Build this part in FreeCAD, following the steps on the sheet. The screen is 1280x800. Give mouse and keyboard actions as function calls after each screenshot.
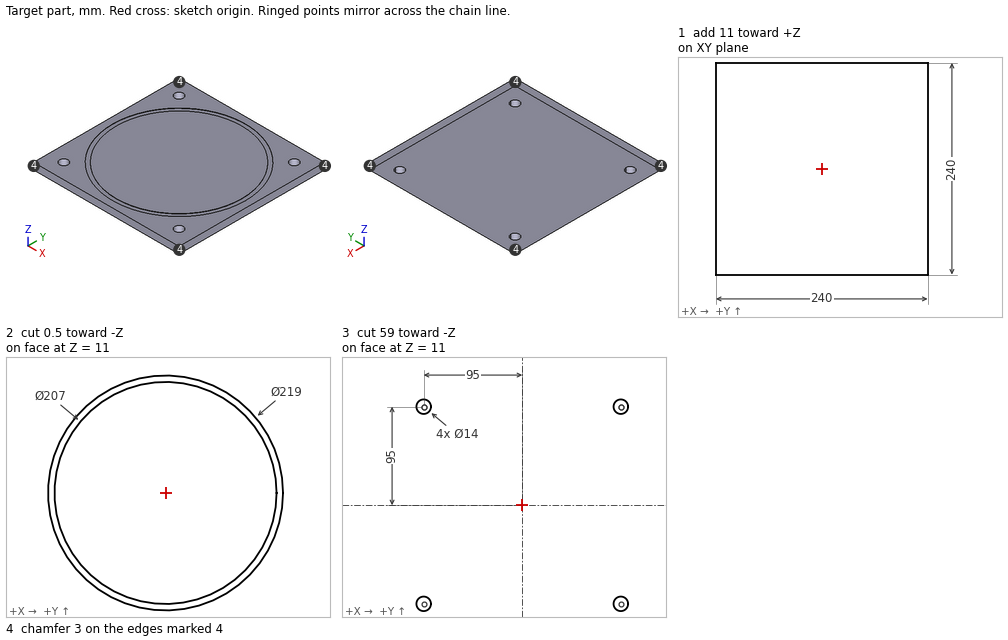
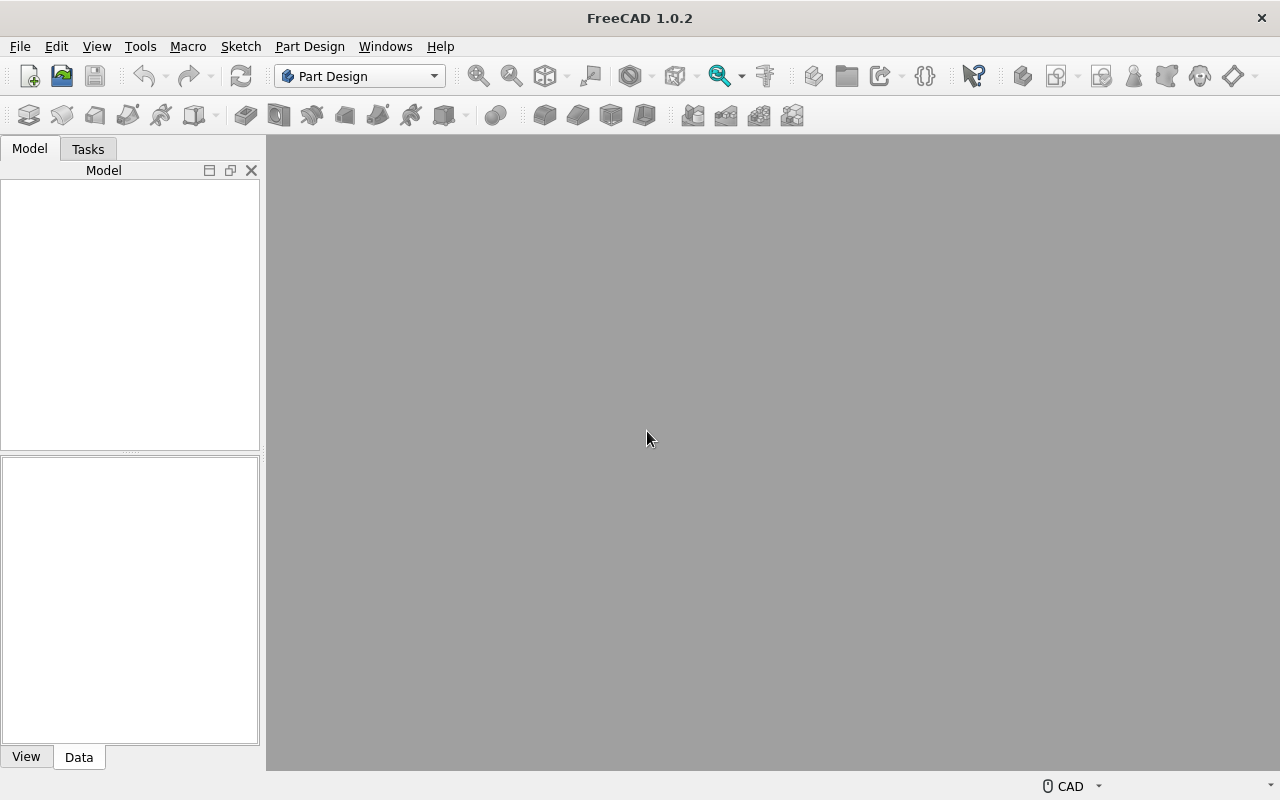
click(29, 76)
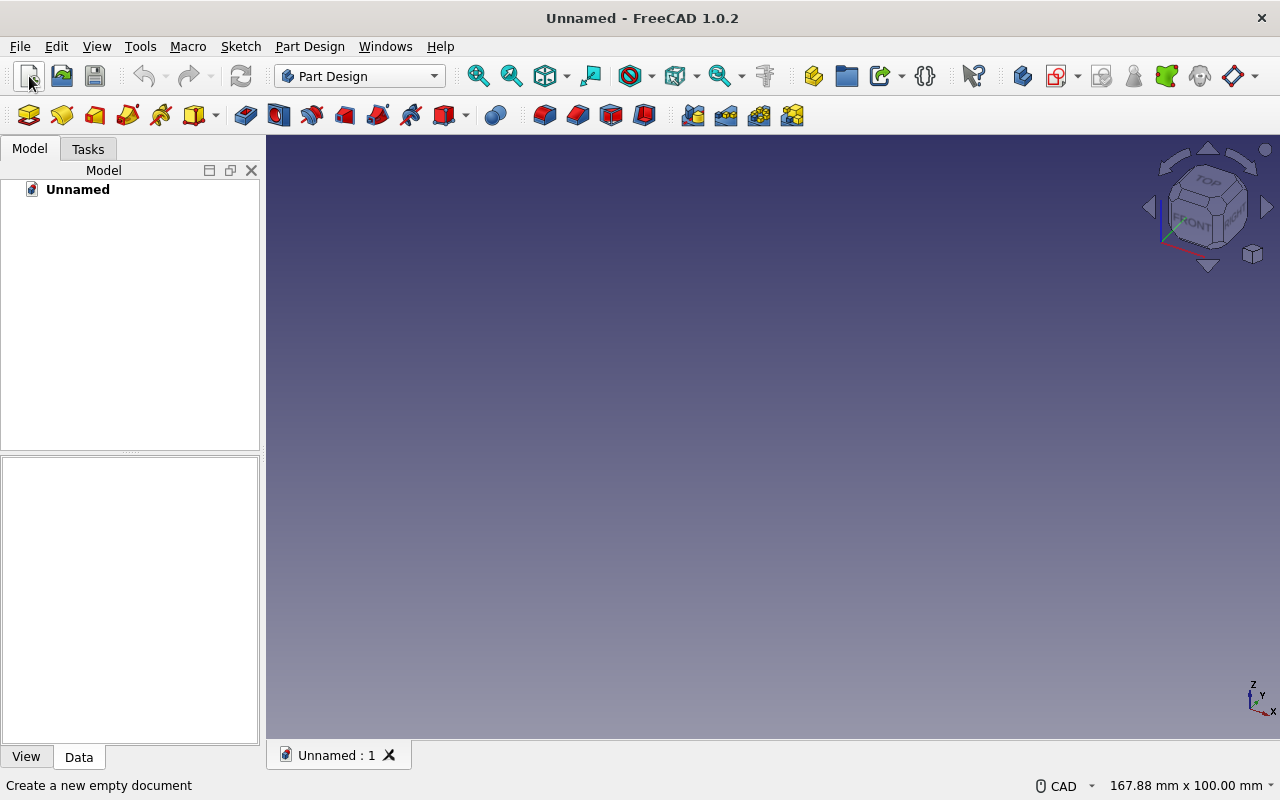
click(1056, 76)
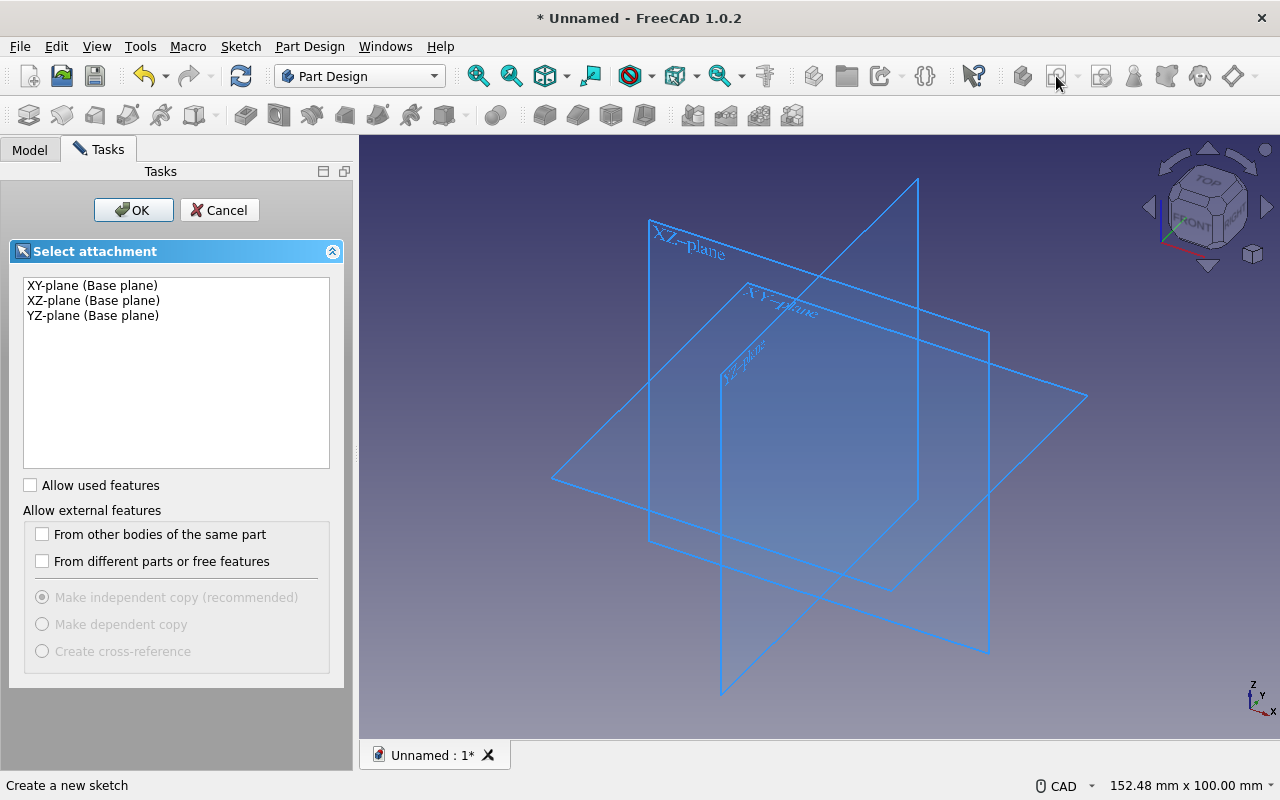
click(84, 286)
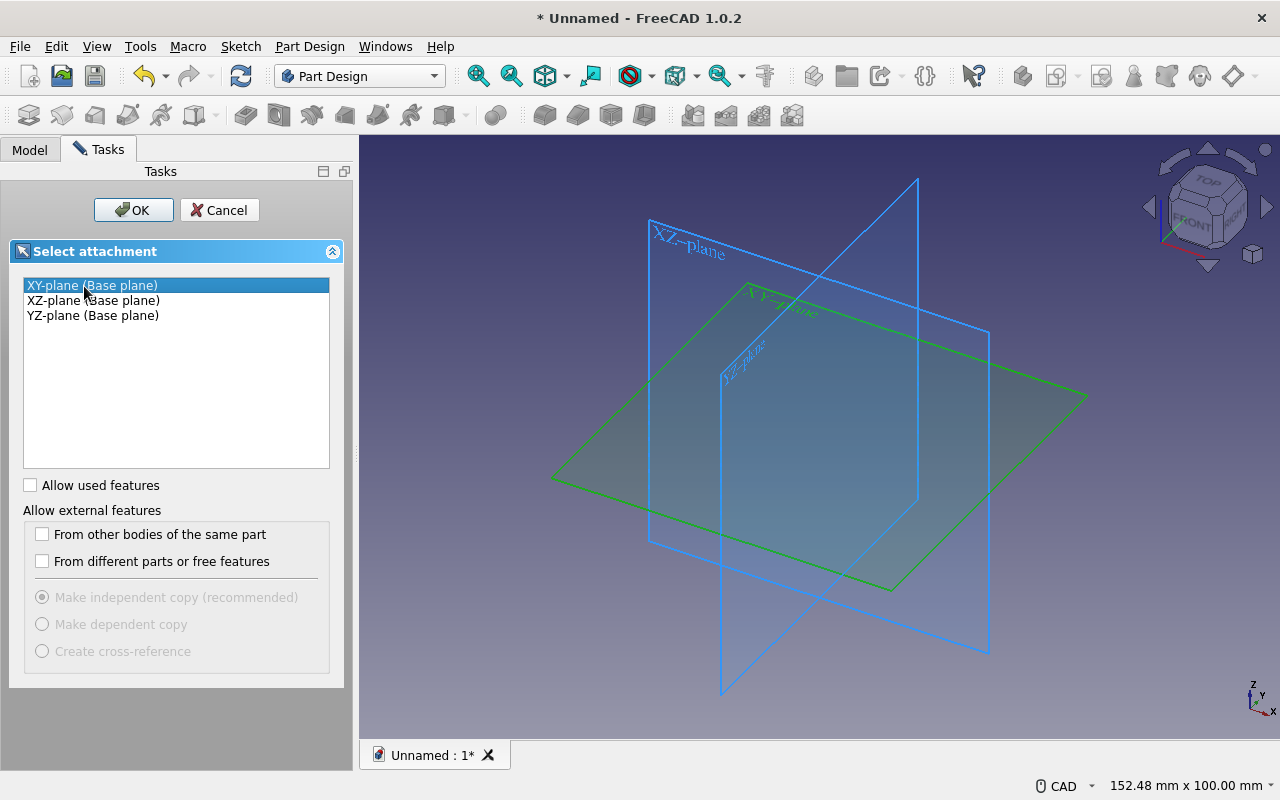
click(134, 210)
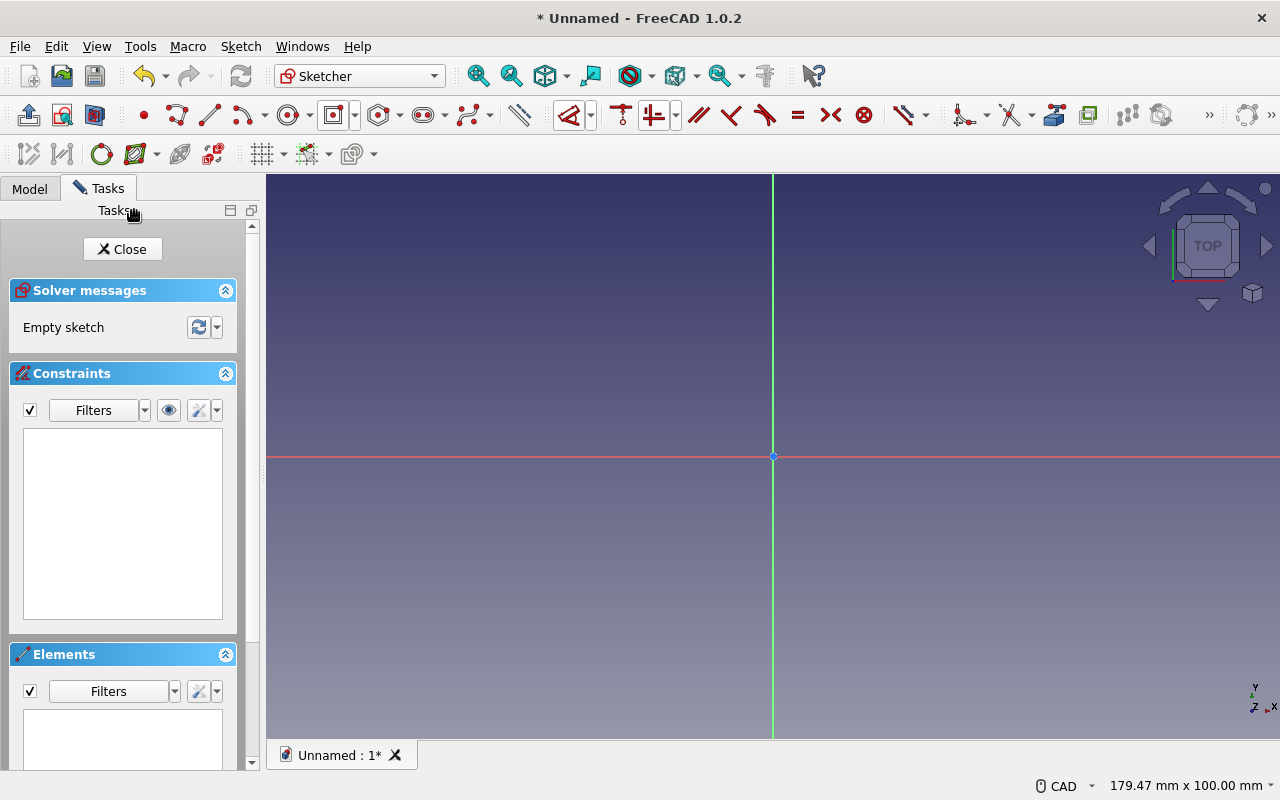
scroll(682, 456, down, 7)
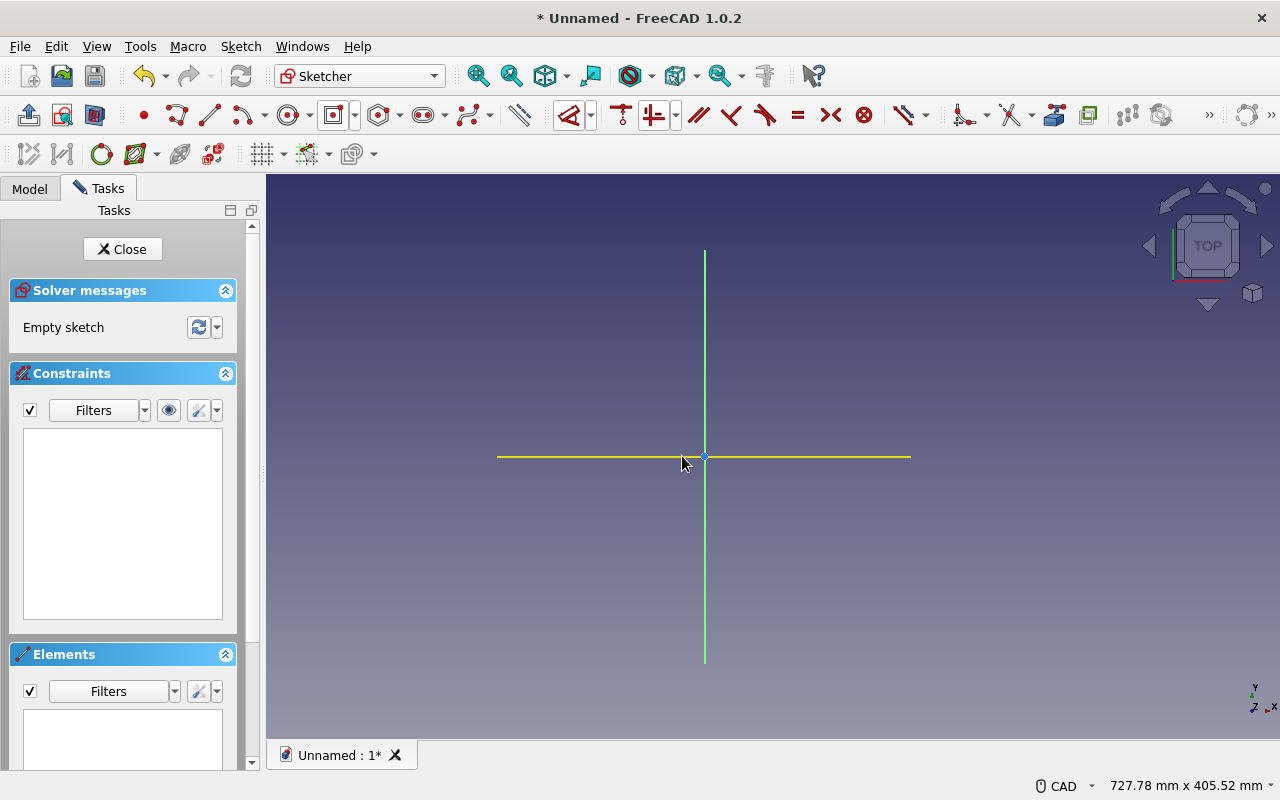
click(332, 116)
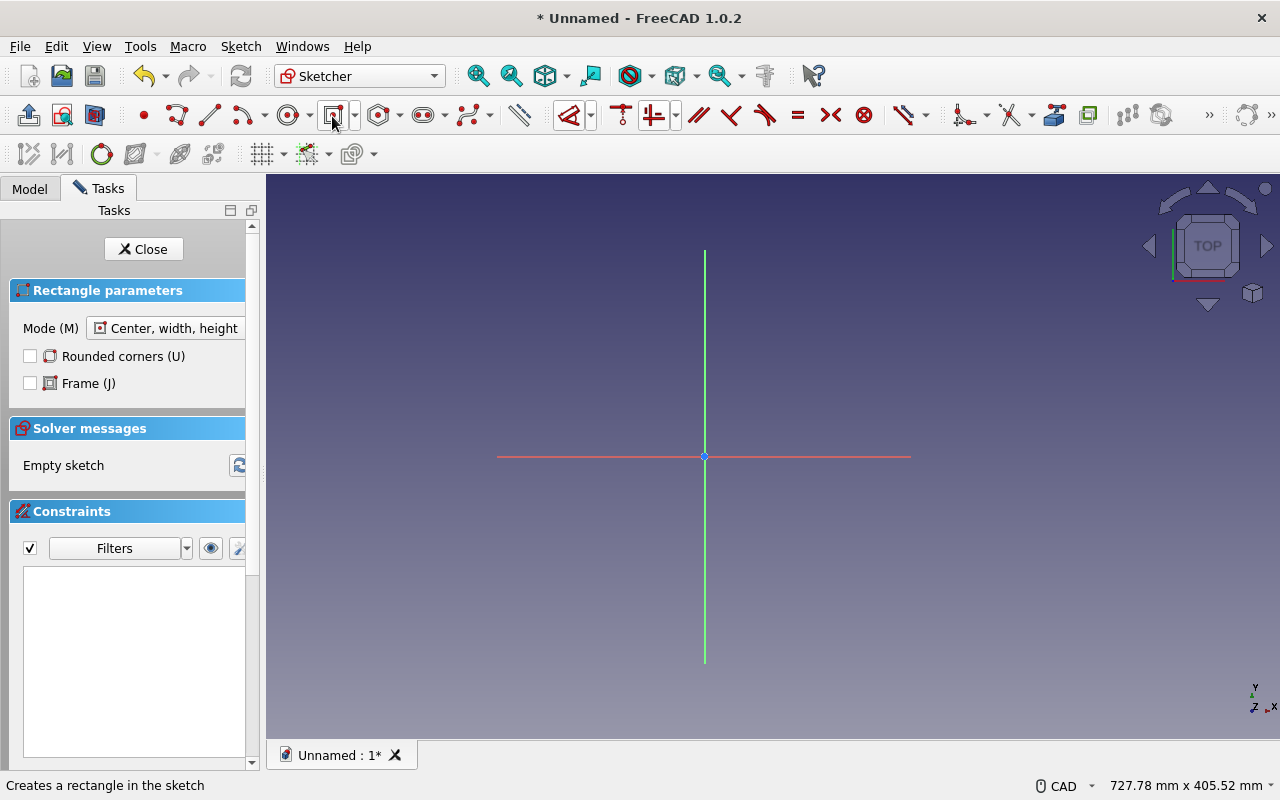
click(705, 456)
move(872, 289)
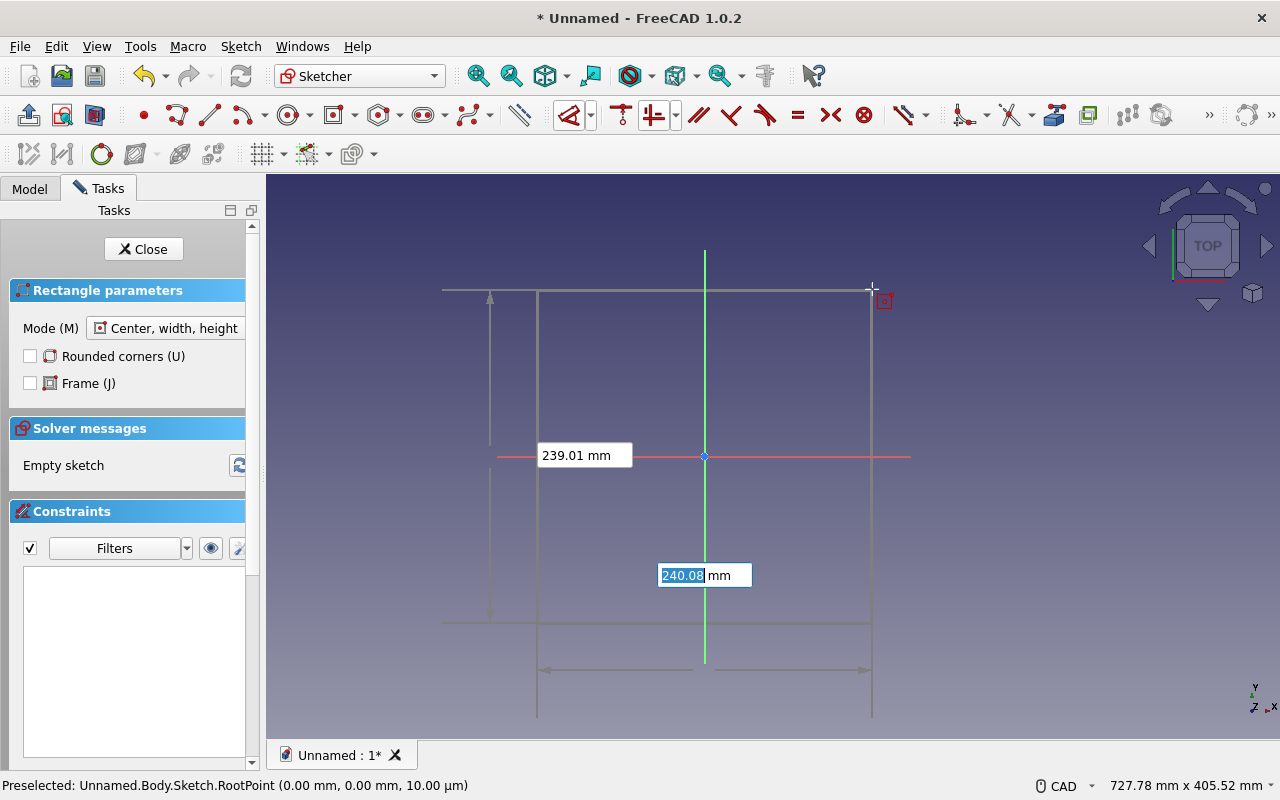
text(240)
key(Tab)
text(240)
key(Return)
key(Escape)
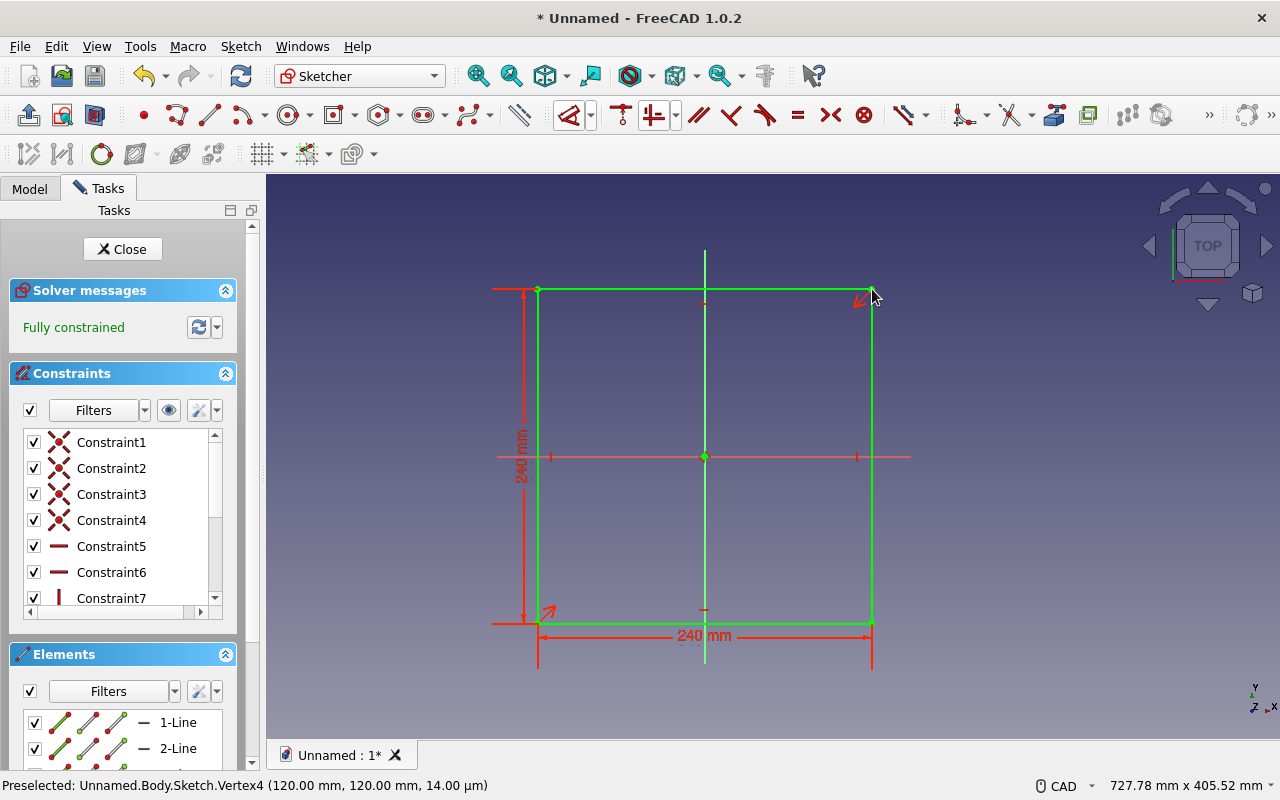
click(123, 249)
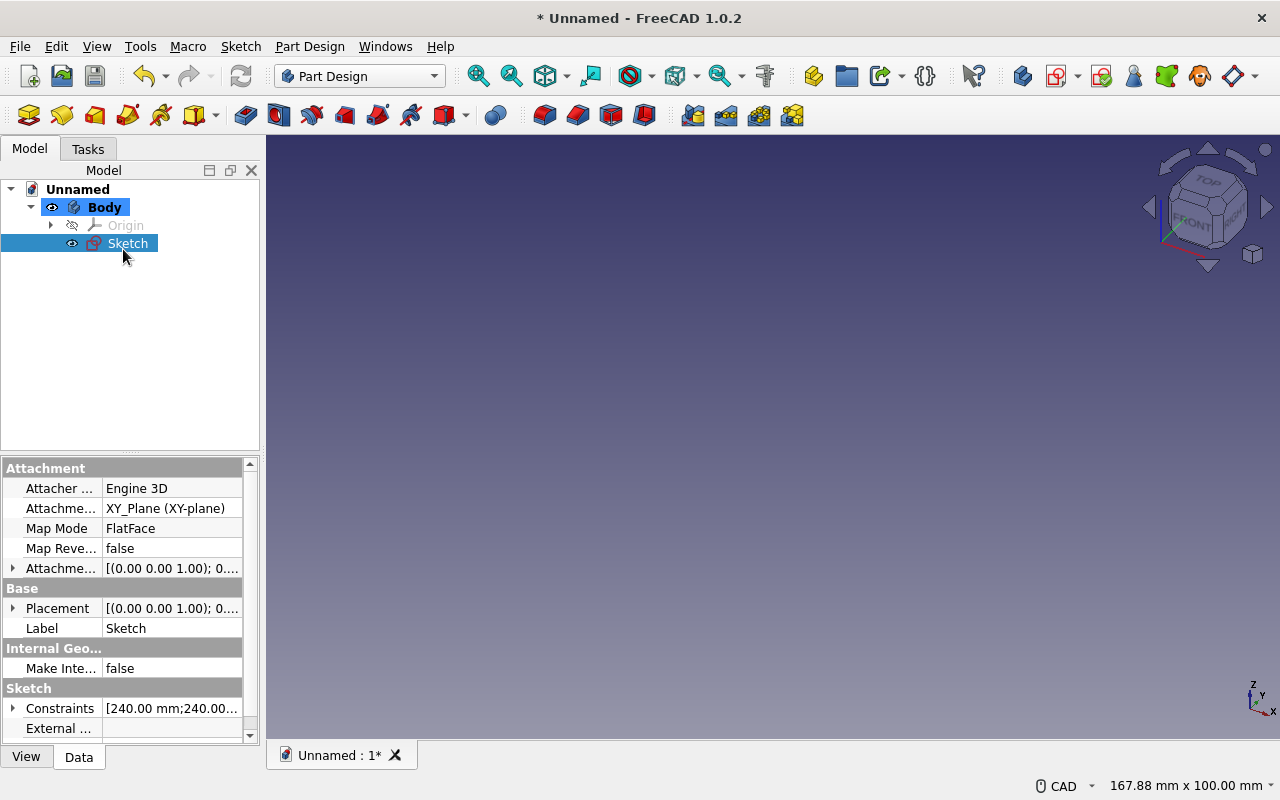
click(29, 116)